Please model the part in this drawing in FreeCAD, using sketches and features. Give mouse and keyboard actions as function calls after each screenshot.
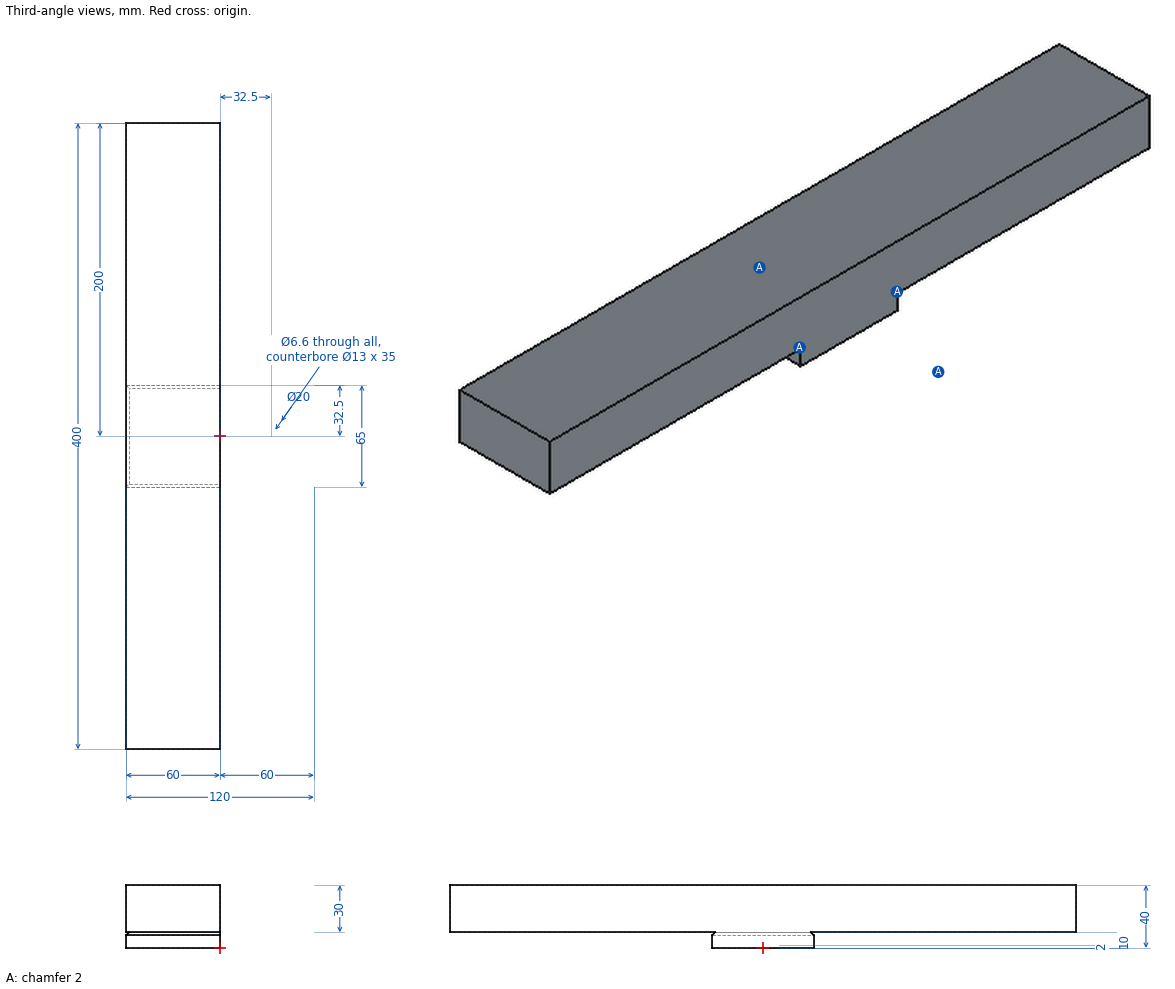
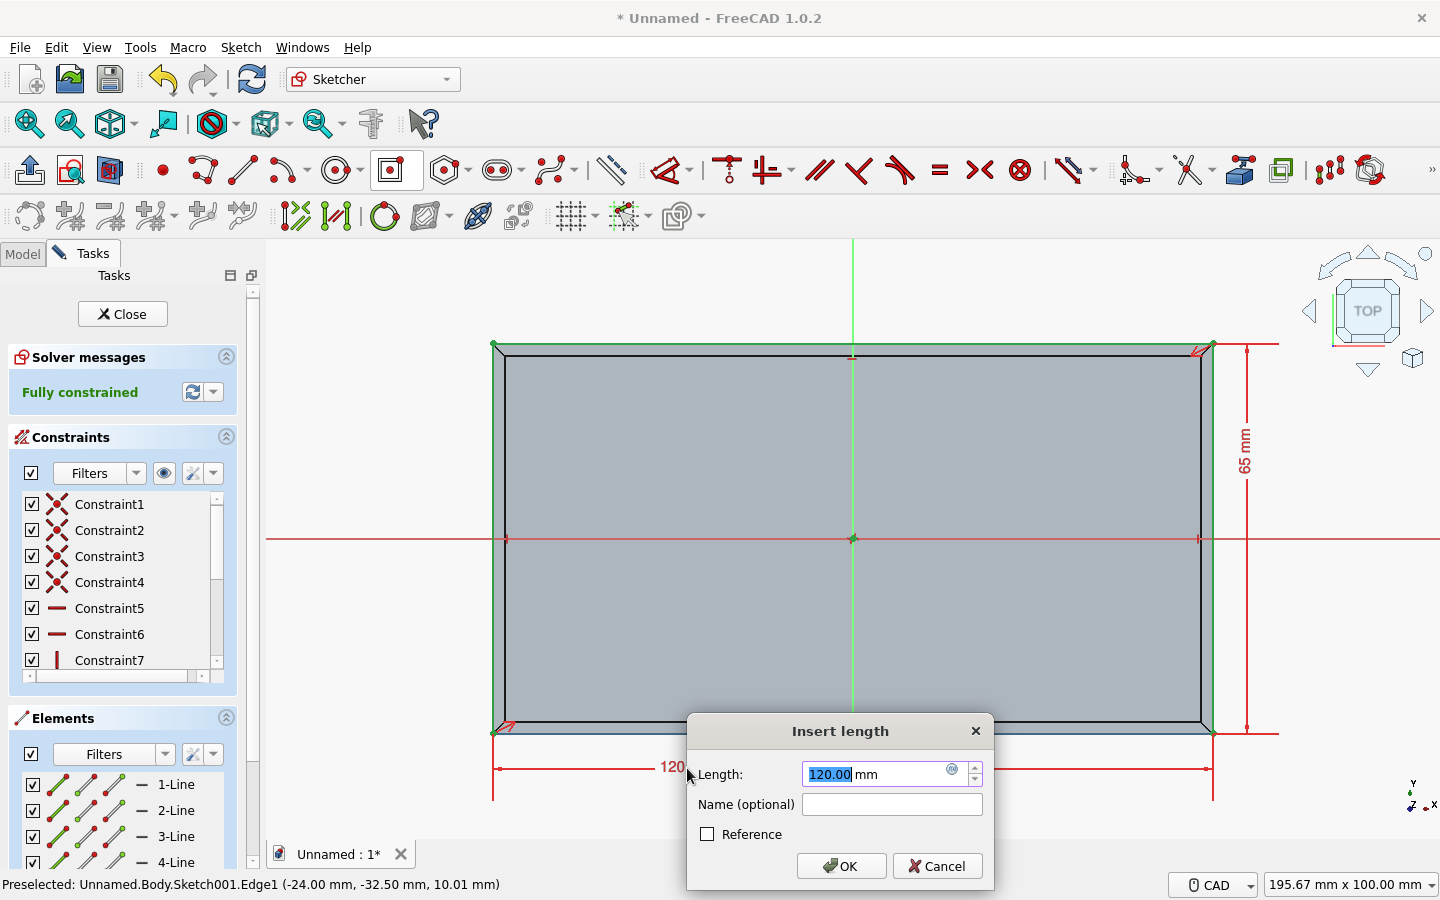
text(120)
key(Return)
key(Escape)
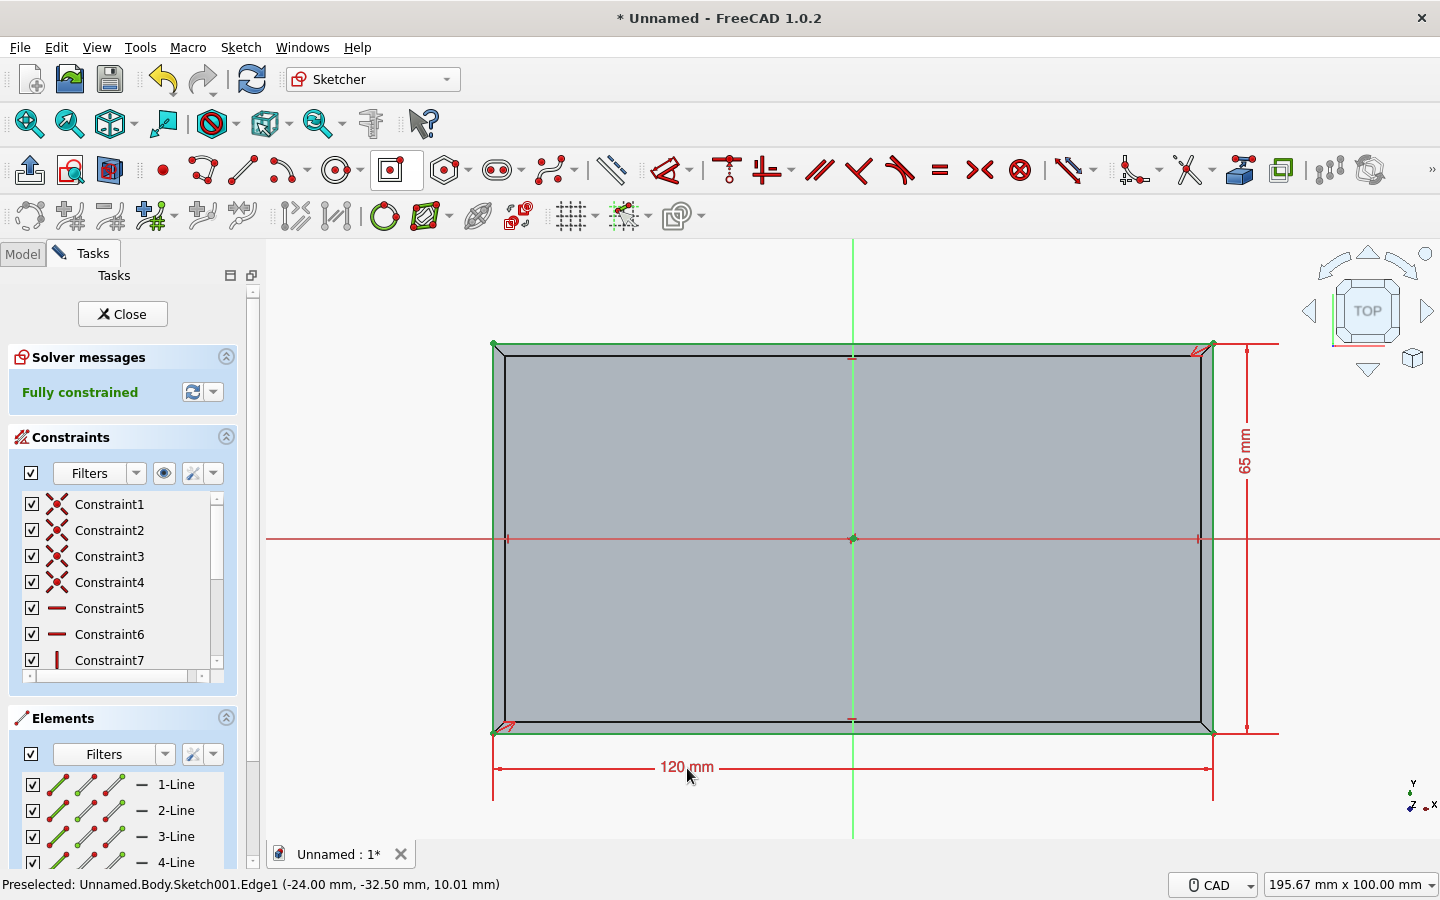
click(123, 314)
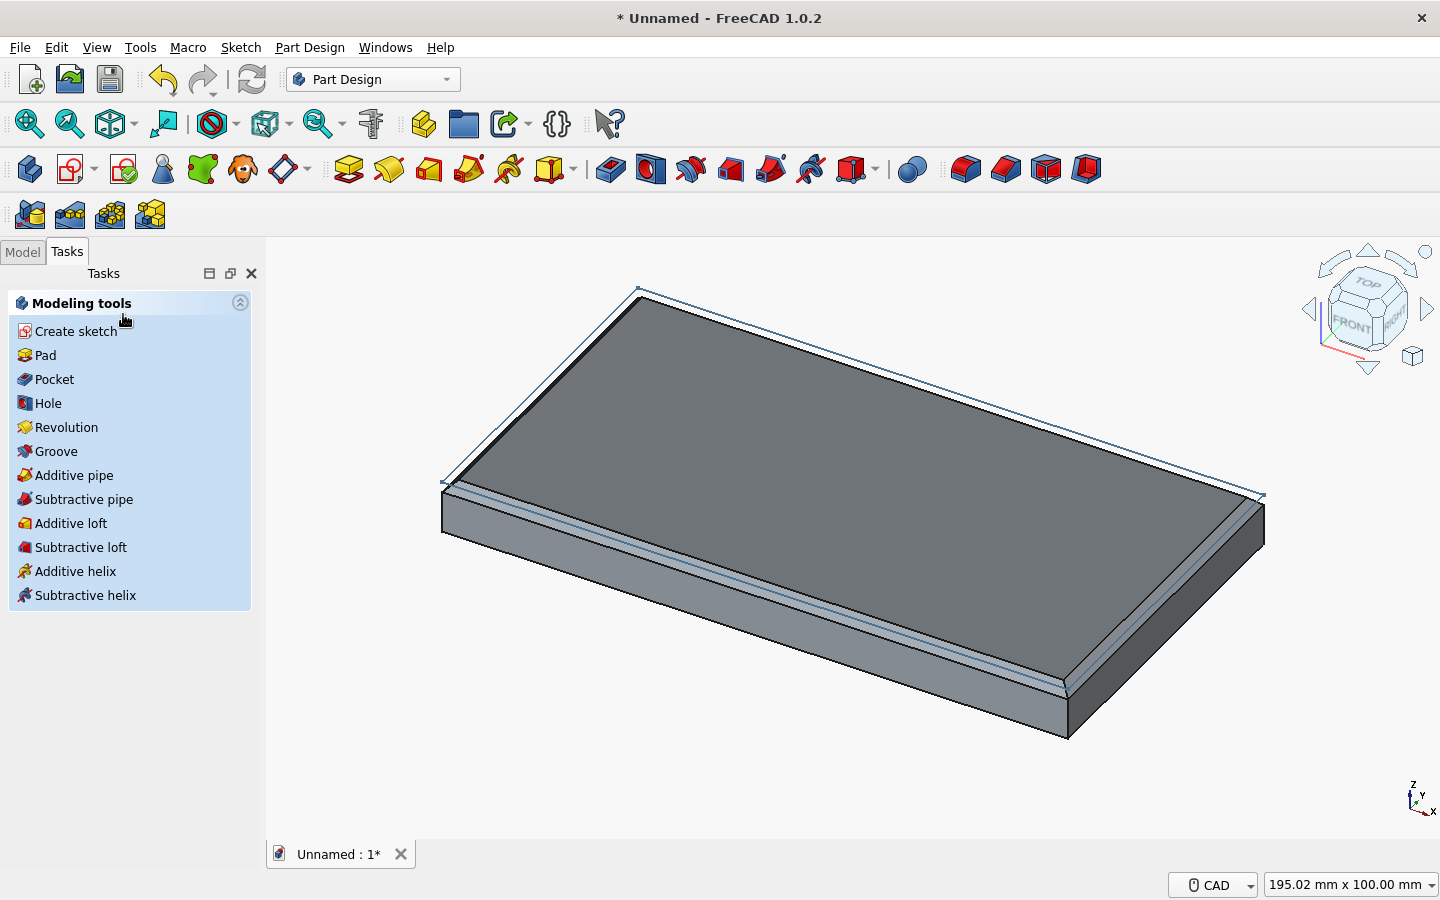
click(350, 170)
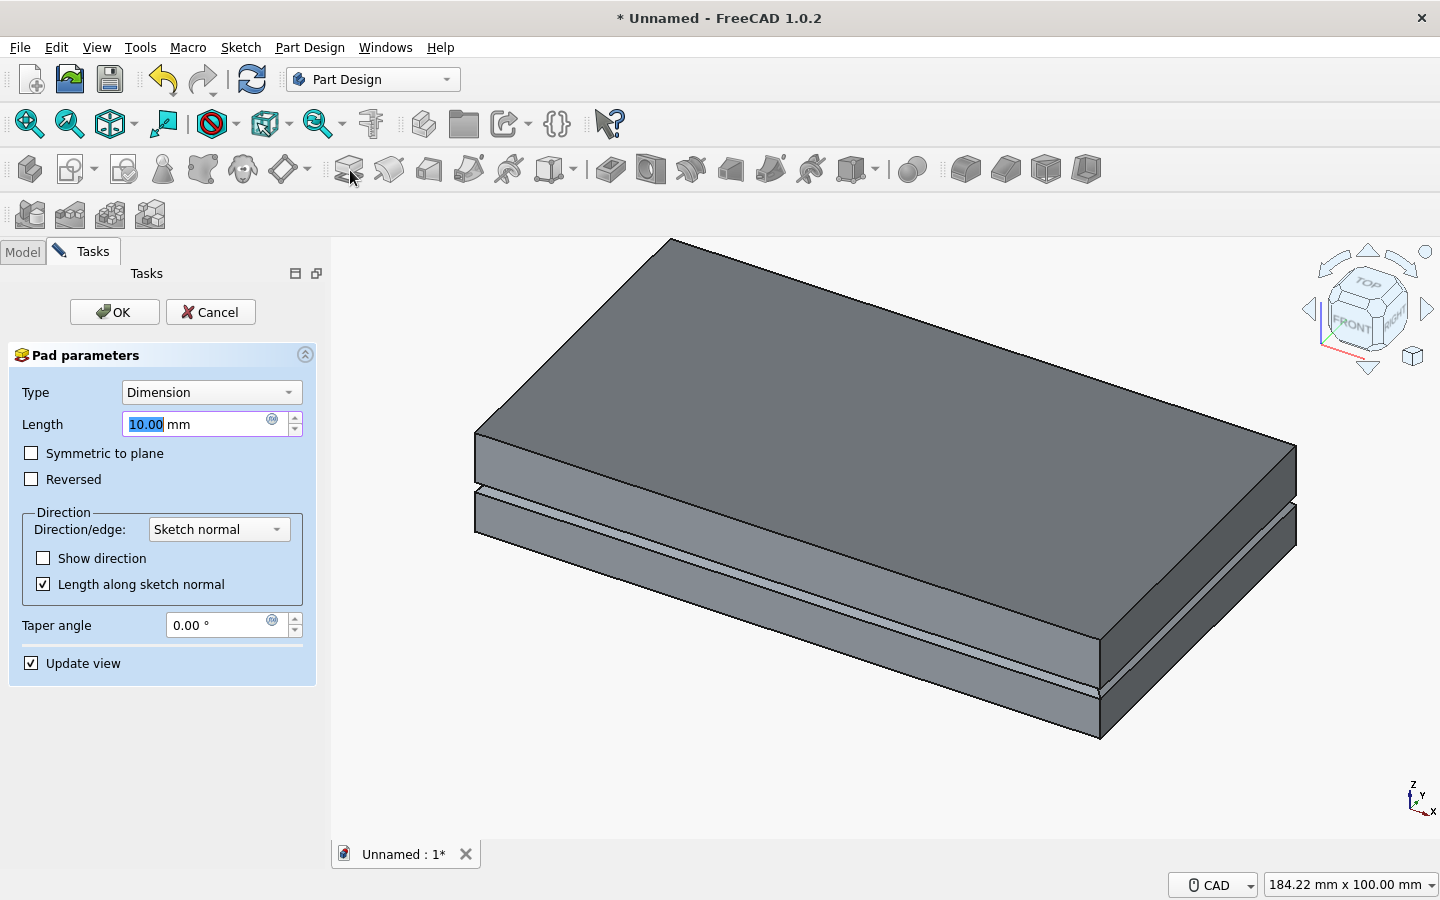
text(30)
key(Tab)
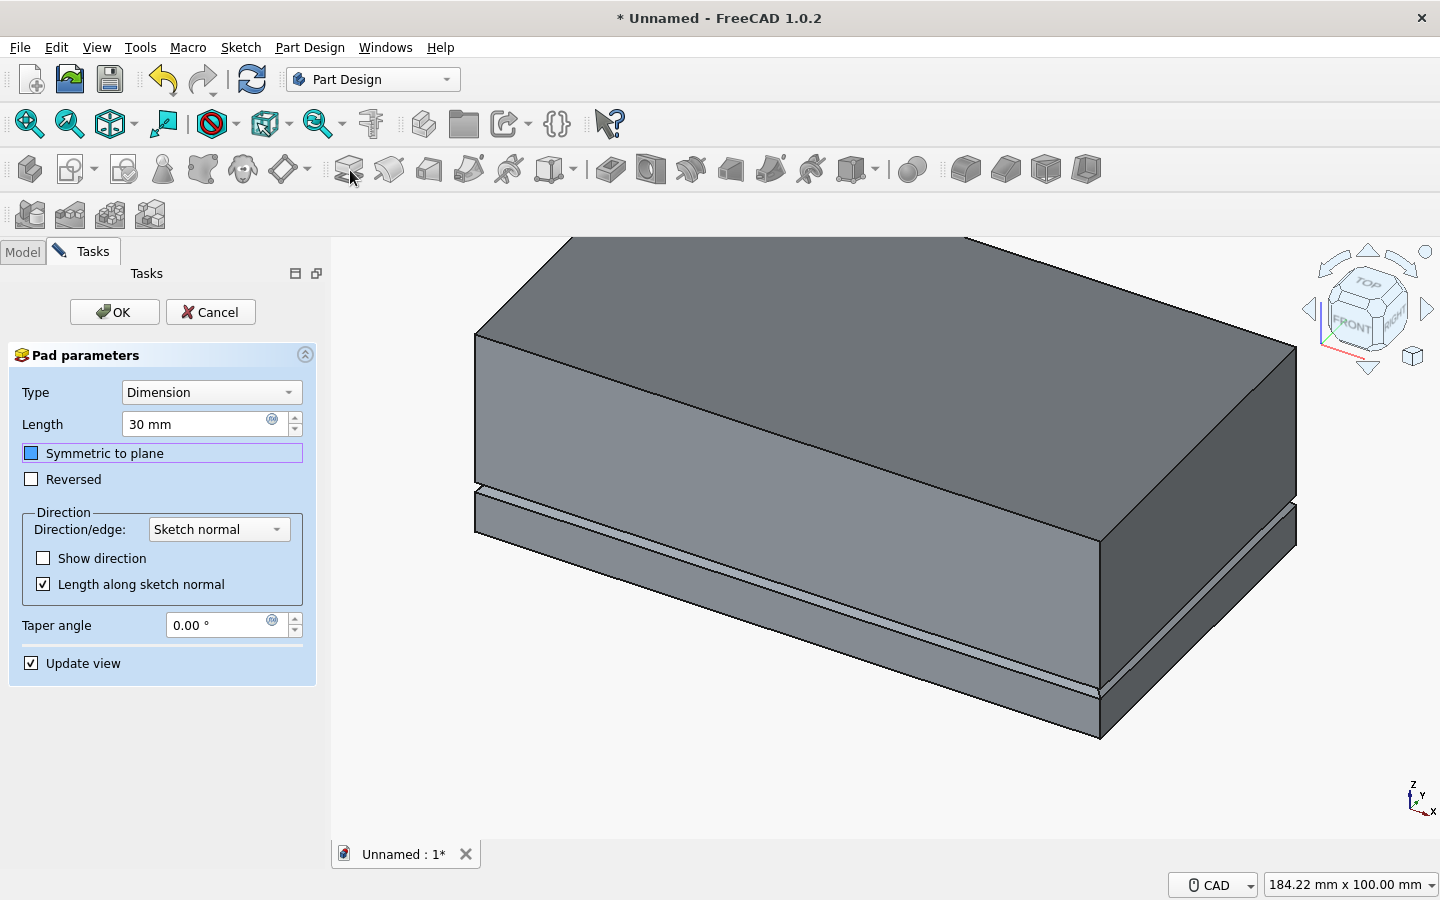
click(115, 312)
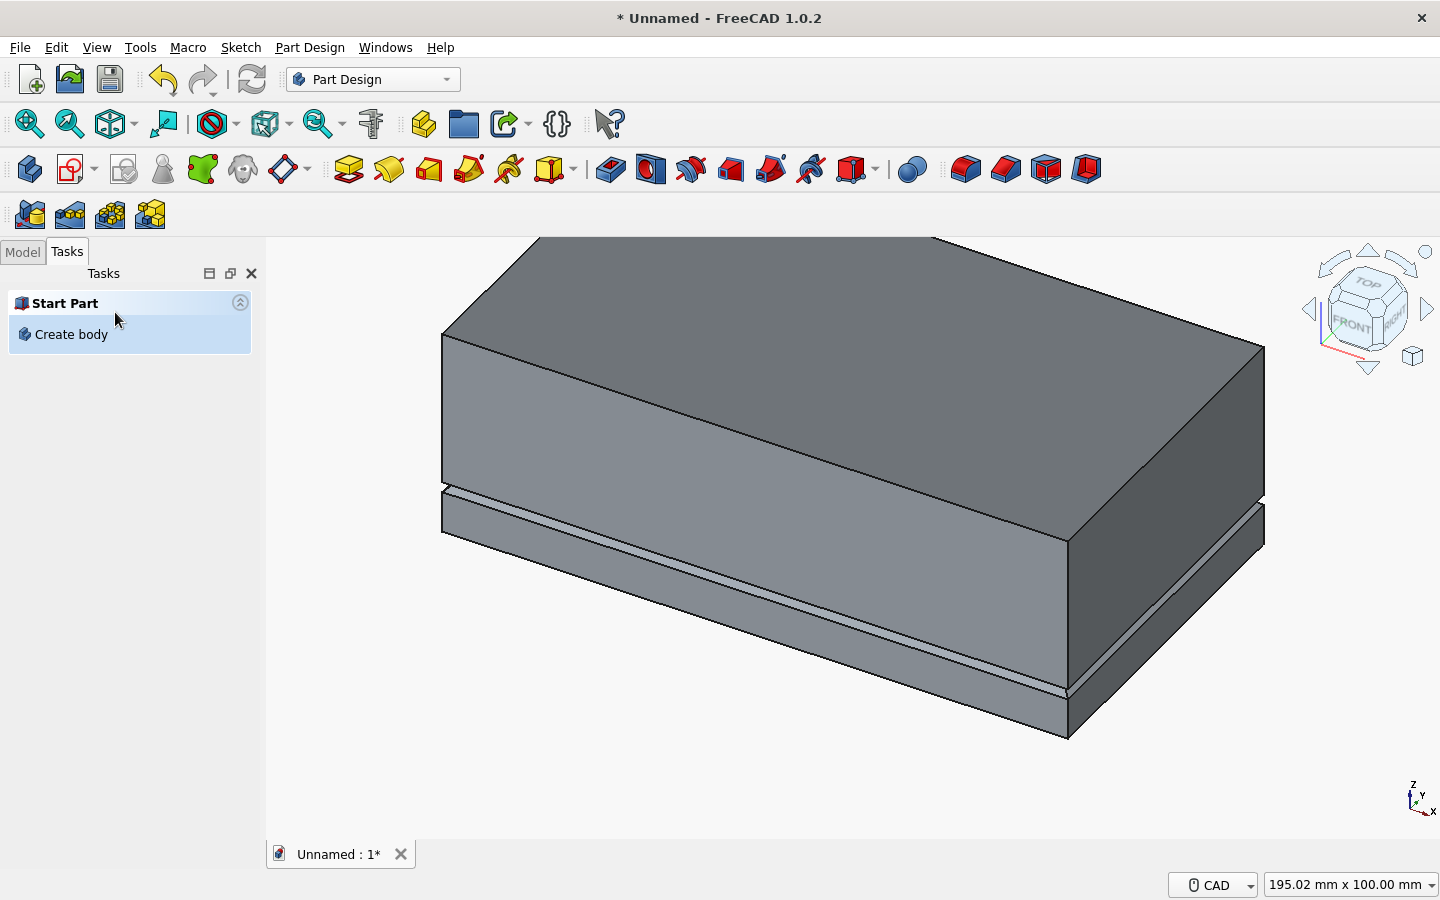
key(v)
key(f)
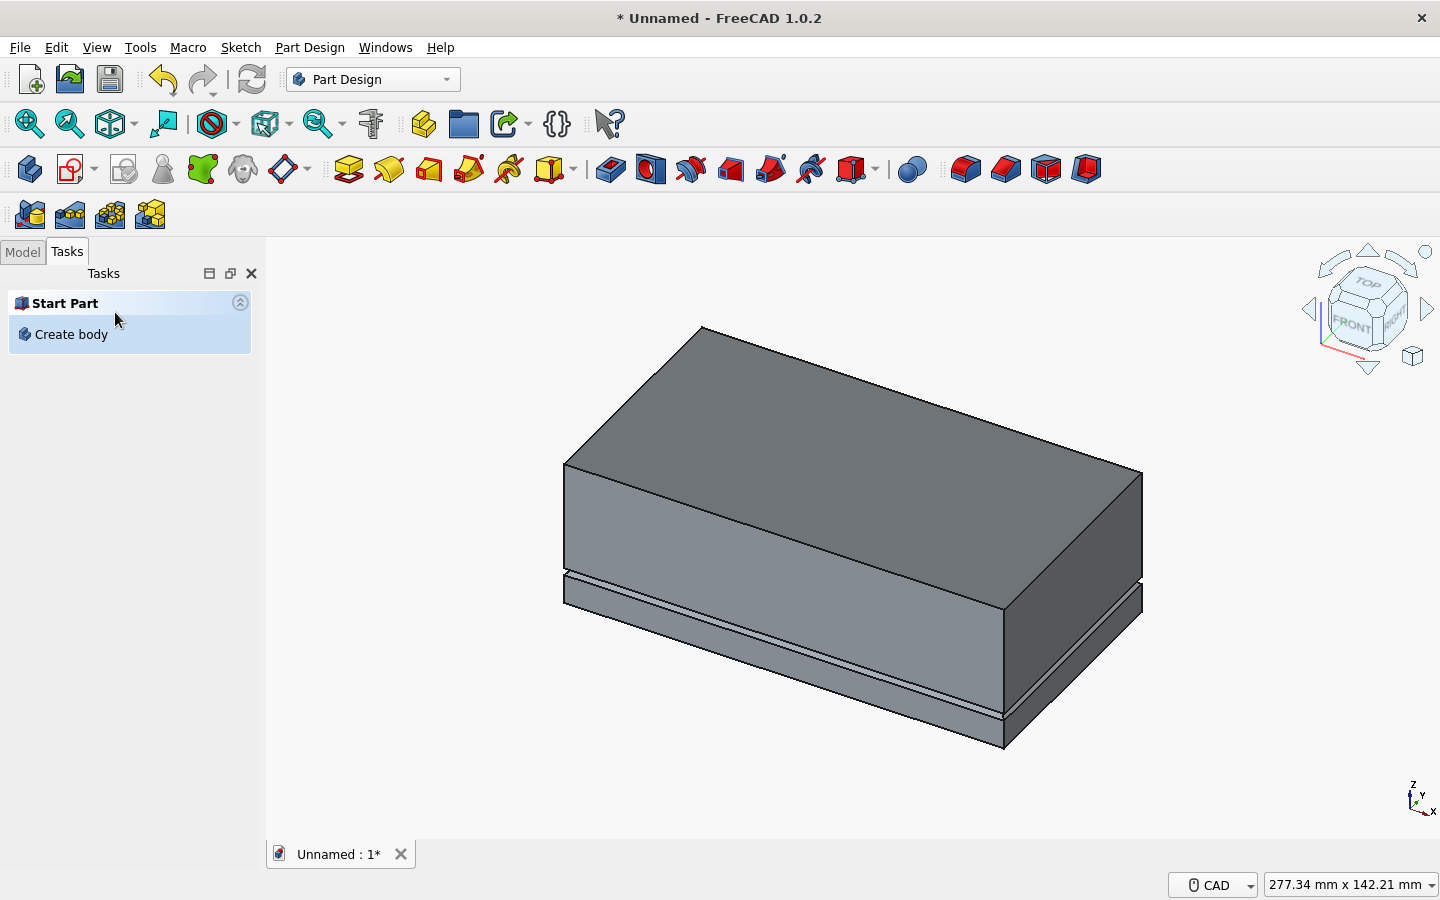
click(70, 170)